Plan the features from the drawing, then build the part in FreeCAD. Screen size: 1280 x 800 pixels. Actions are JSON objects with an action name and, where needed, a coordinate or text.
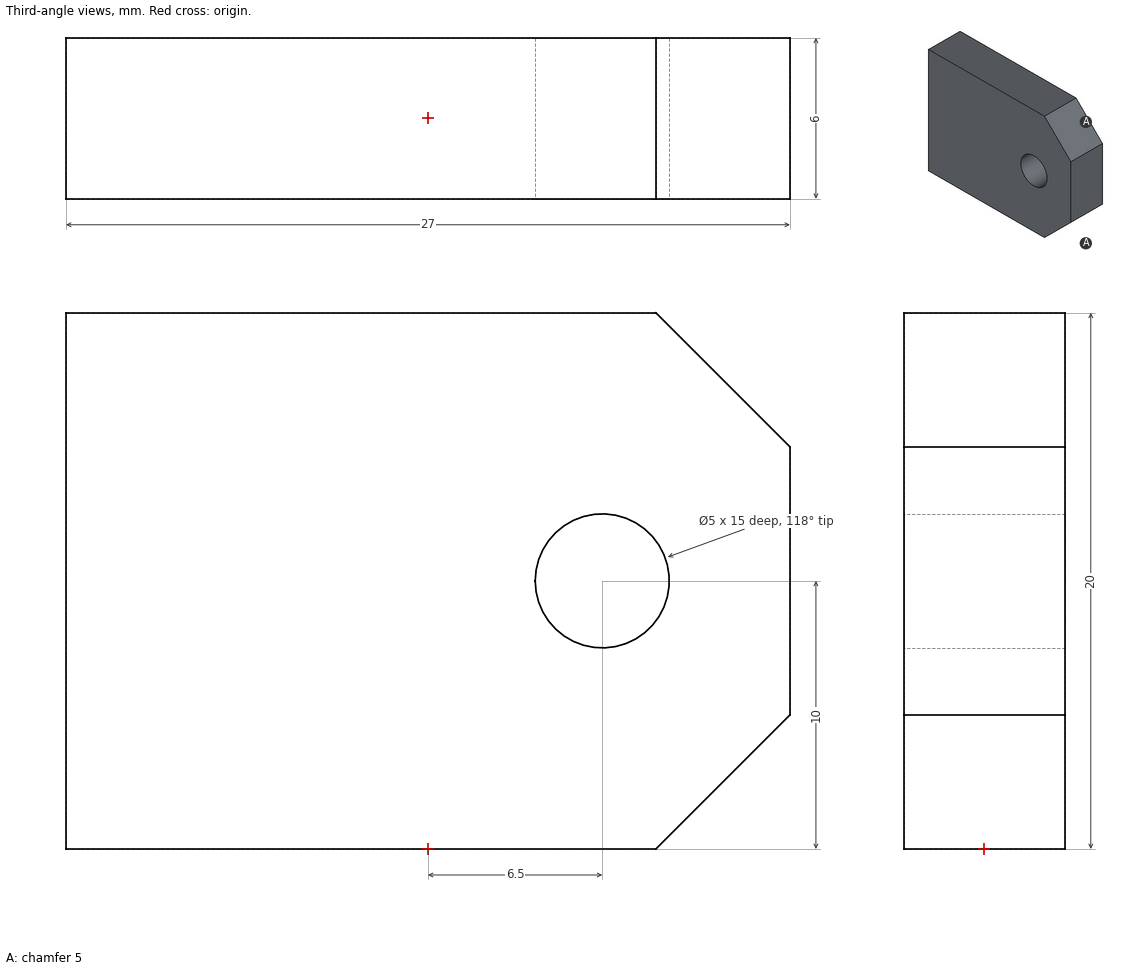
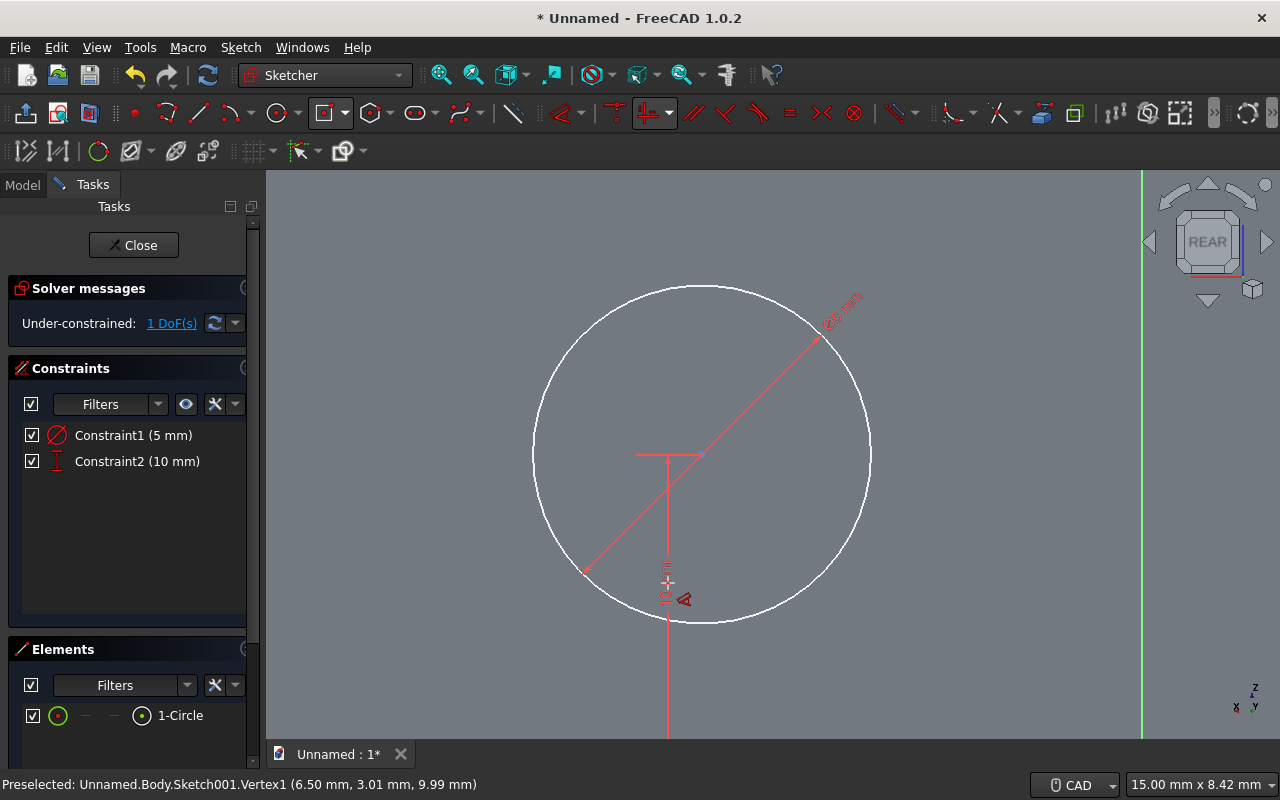
{"action": "left_click", "coordinate": [702, 454]}
{"action": "left_click", "coordinate": [908, 420]}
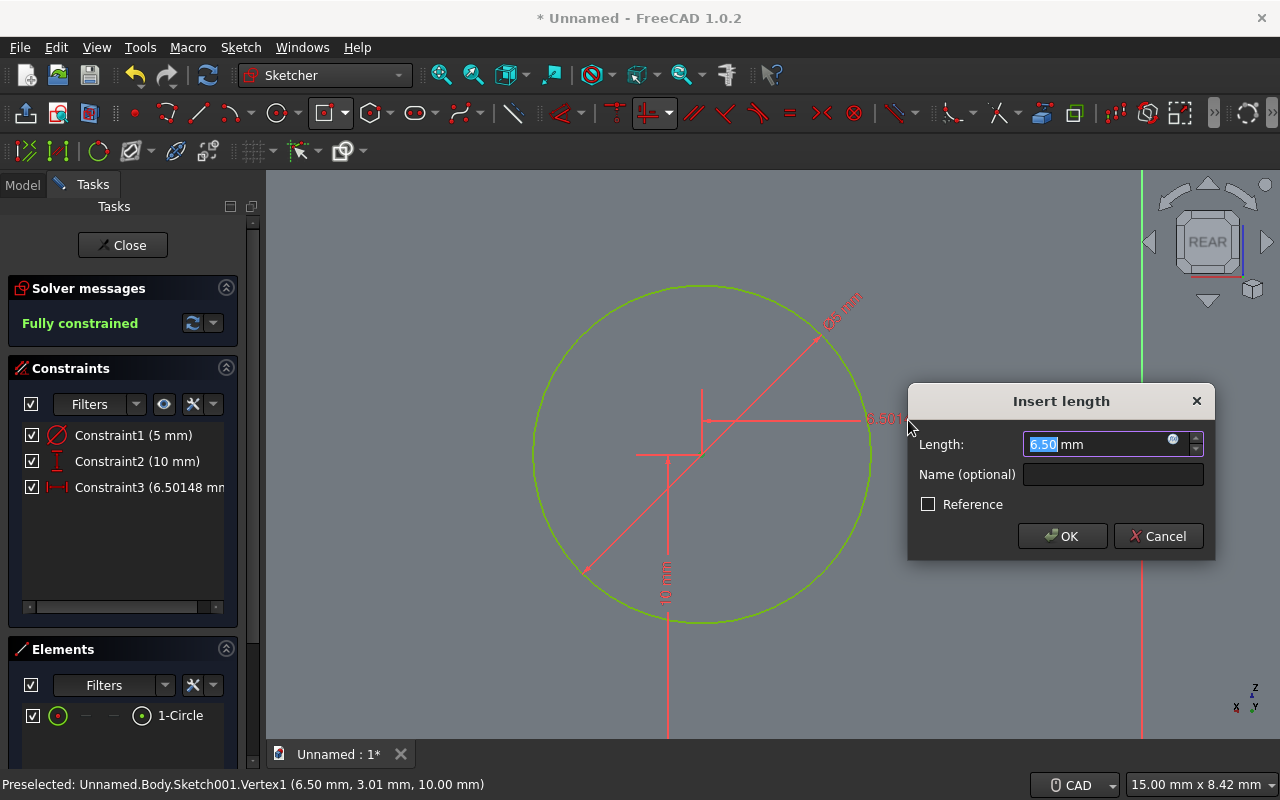
{"action": "type", "text": "6.5"}
{"action": "key", "text": "Return"}
{"action": "key", "text": "Escape"}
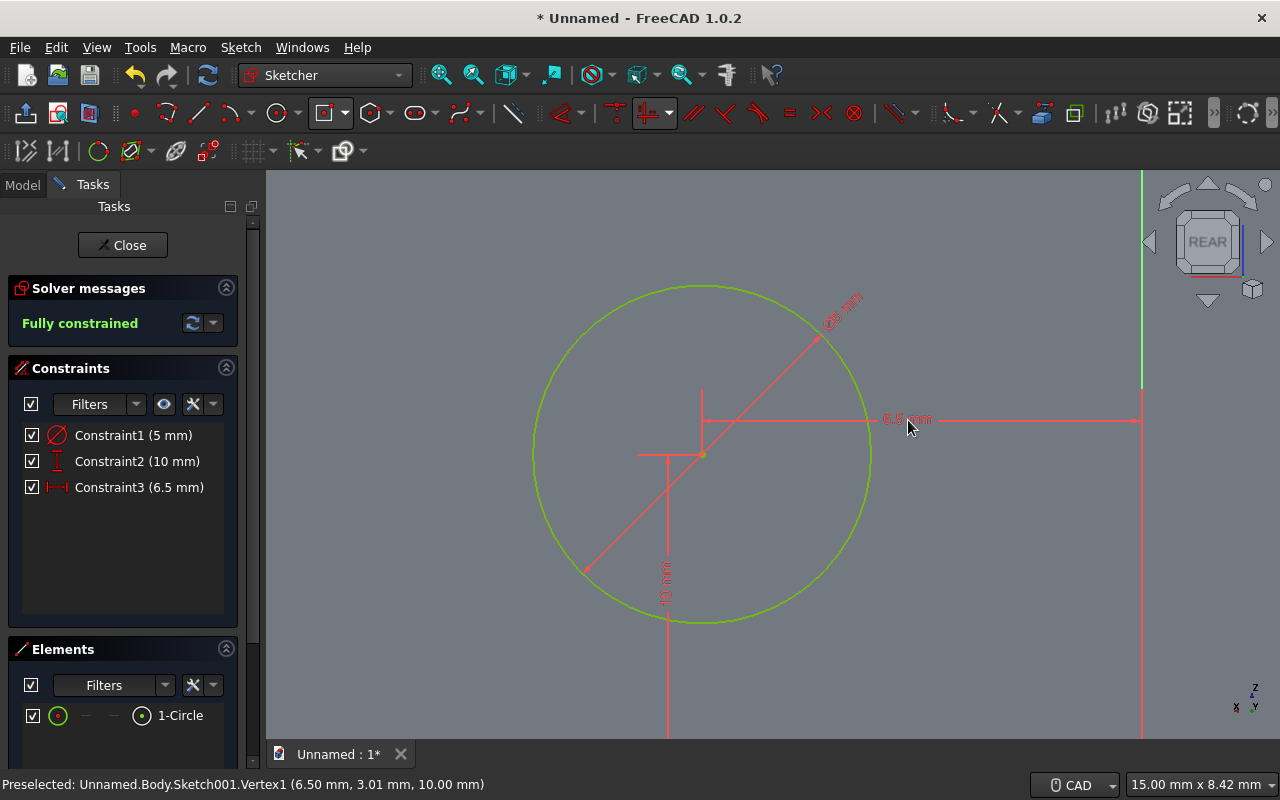
{"action": "left_click", "coordinate": [123, 245]}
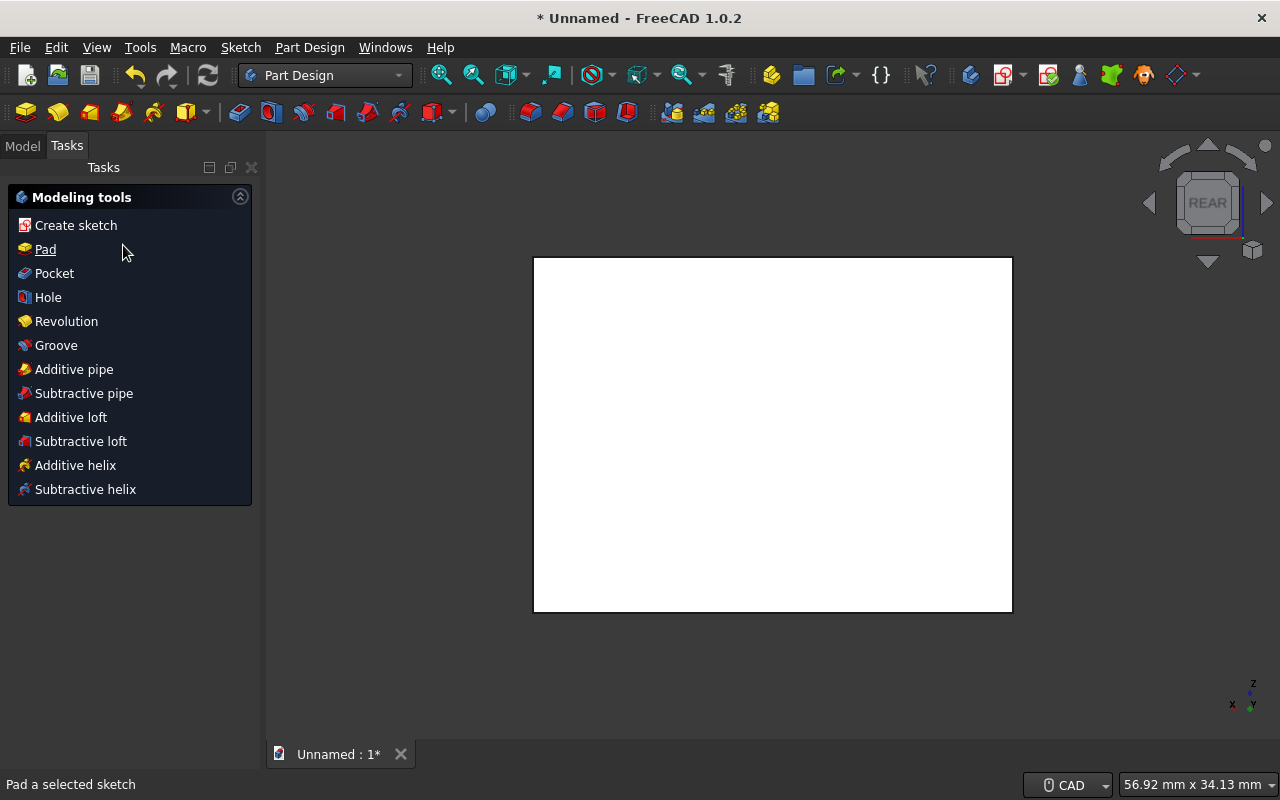
{"action": "left_click", "coordinate": [272, 112]}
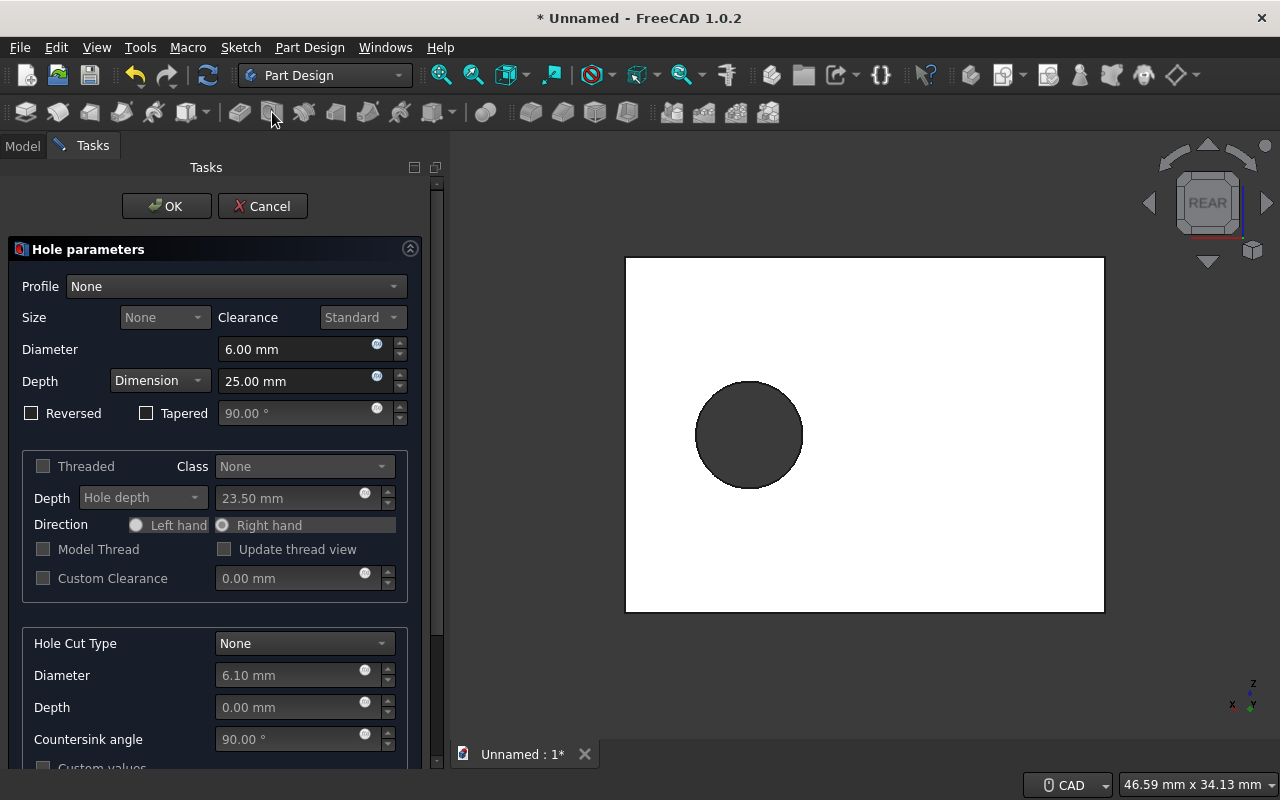
{"action": "triple_click", "coordinate": [305, 349]}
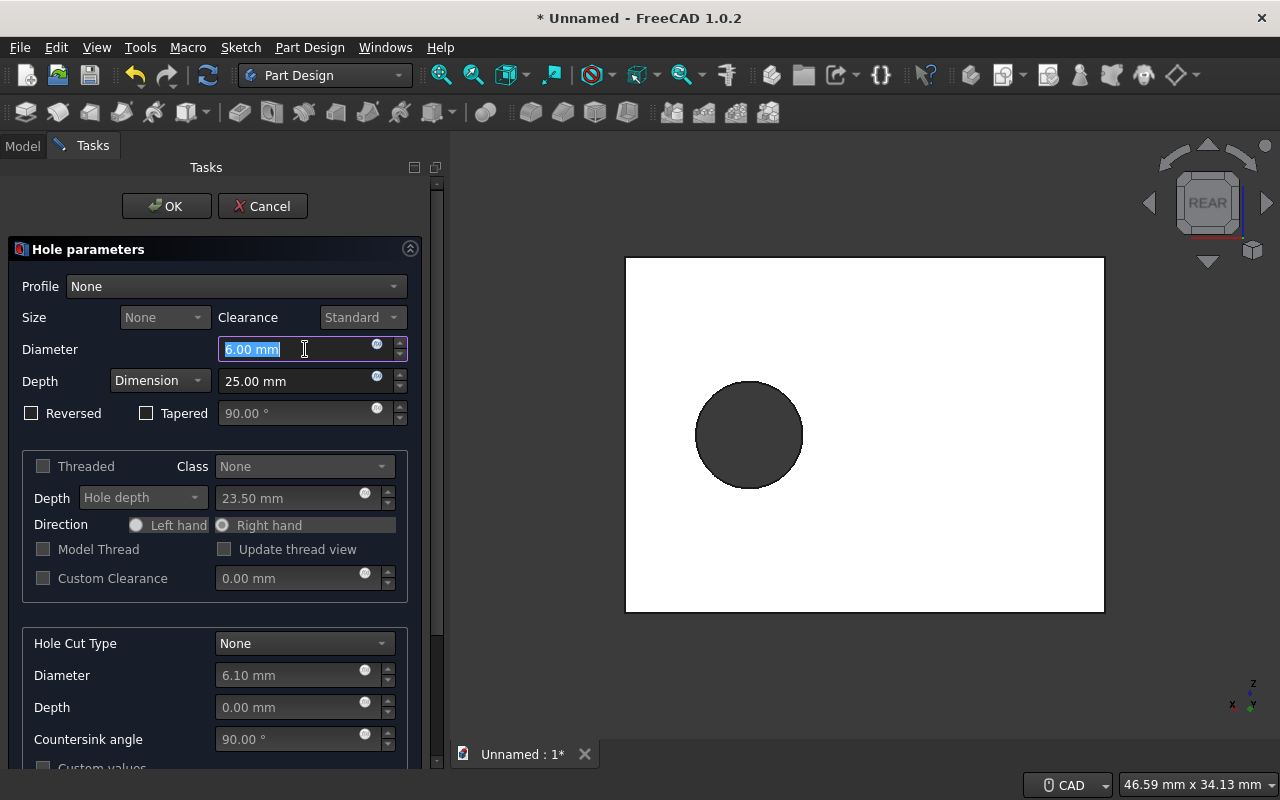
{"action": "type", "text": "5"}
{"action": "key", "text": "Tab"}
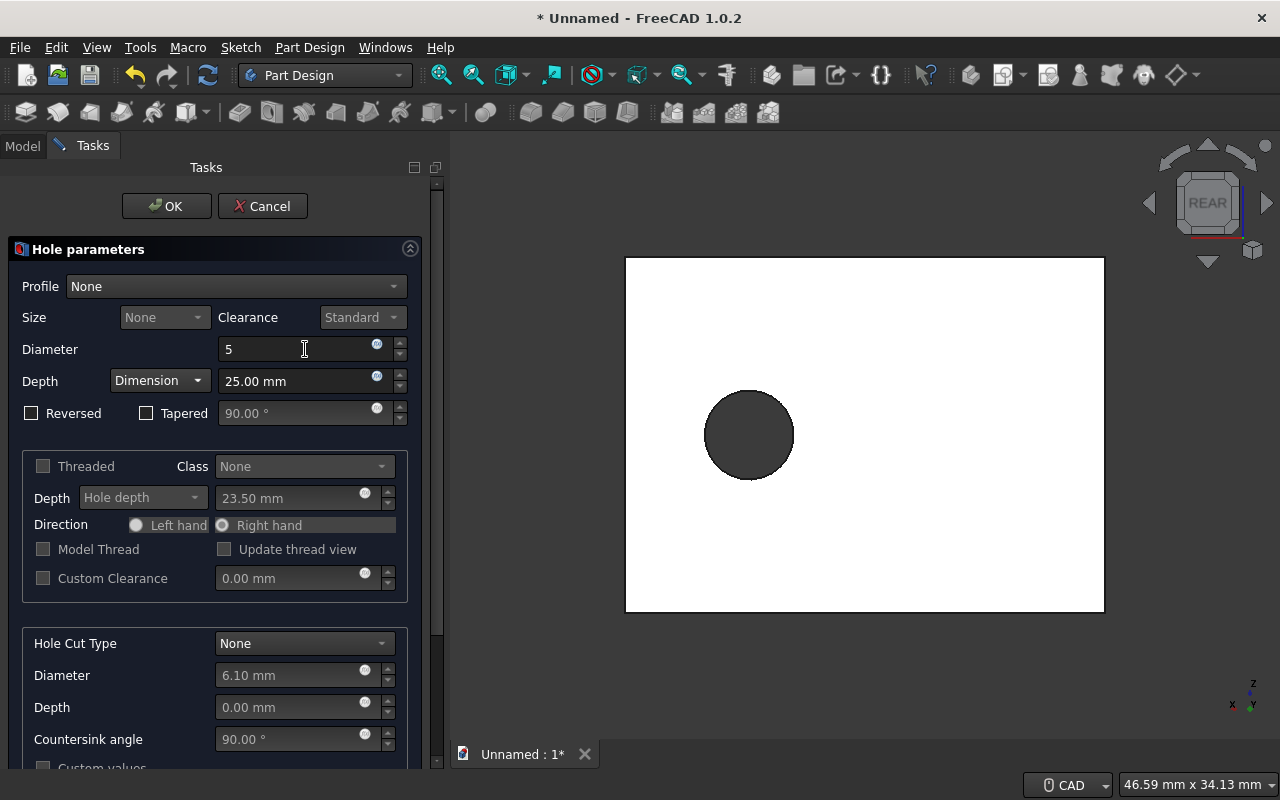
{"action": "triple_click", "coordinate": [305, 381]}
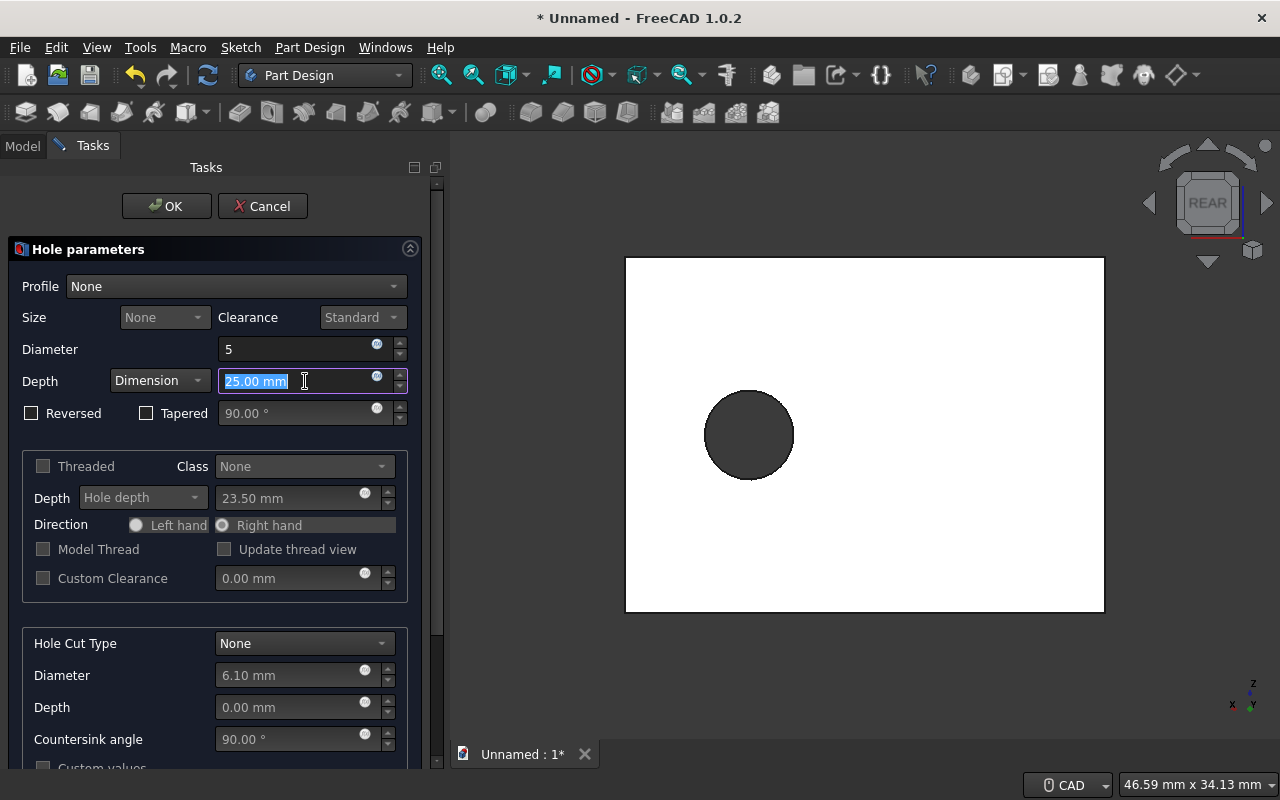
{"action": "type", "text": "15"}
{"action": "key", "text": "Tab"}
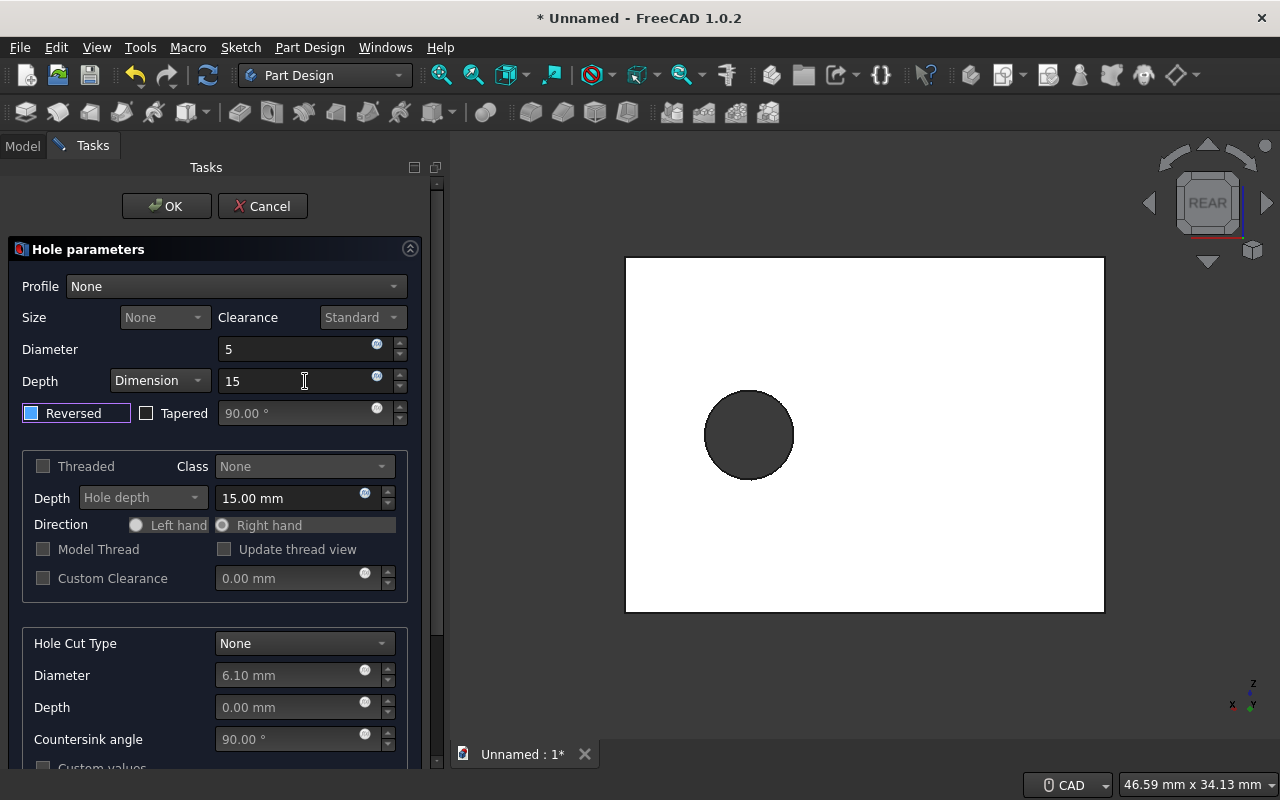
{"action": "left_click", "coordinate": [167, 206]}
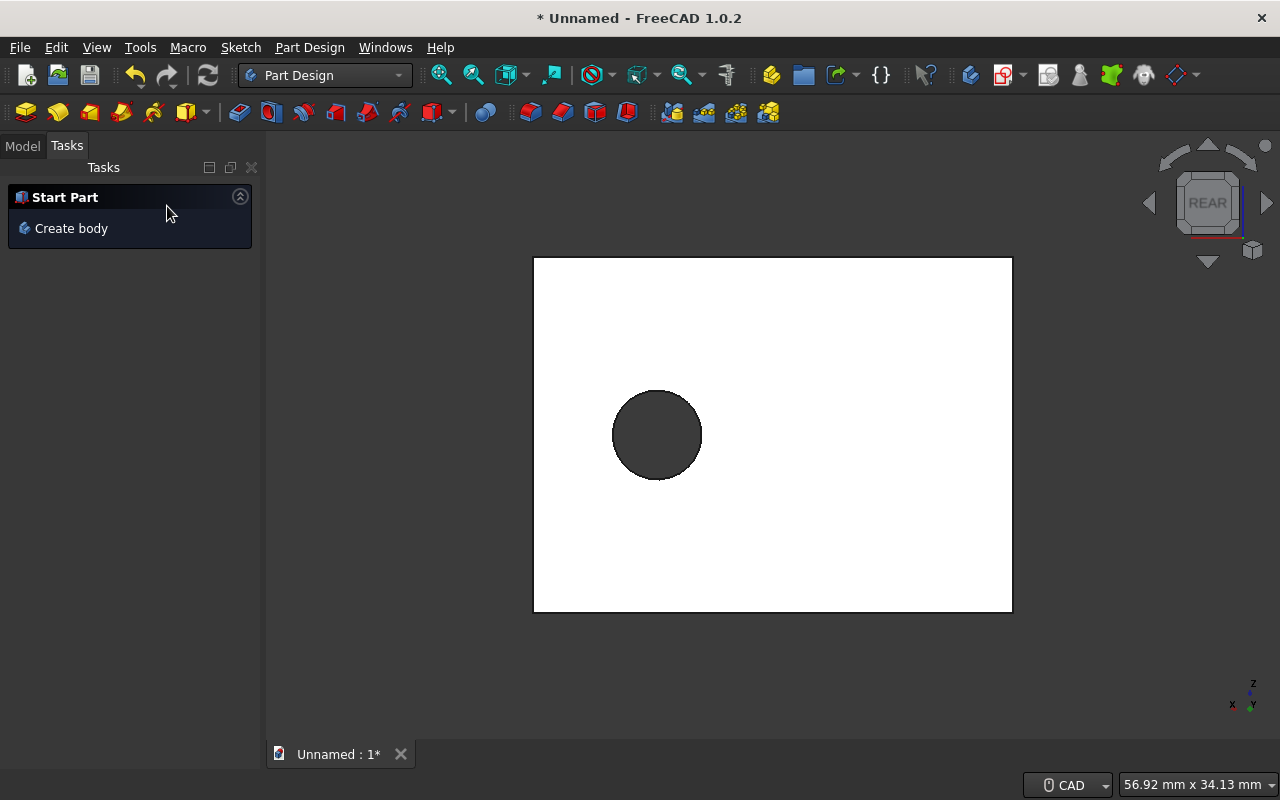
{"action": "key", "text": "0"}